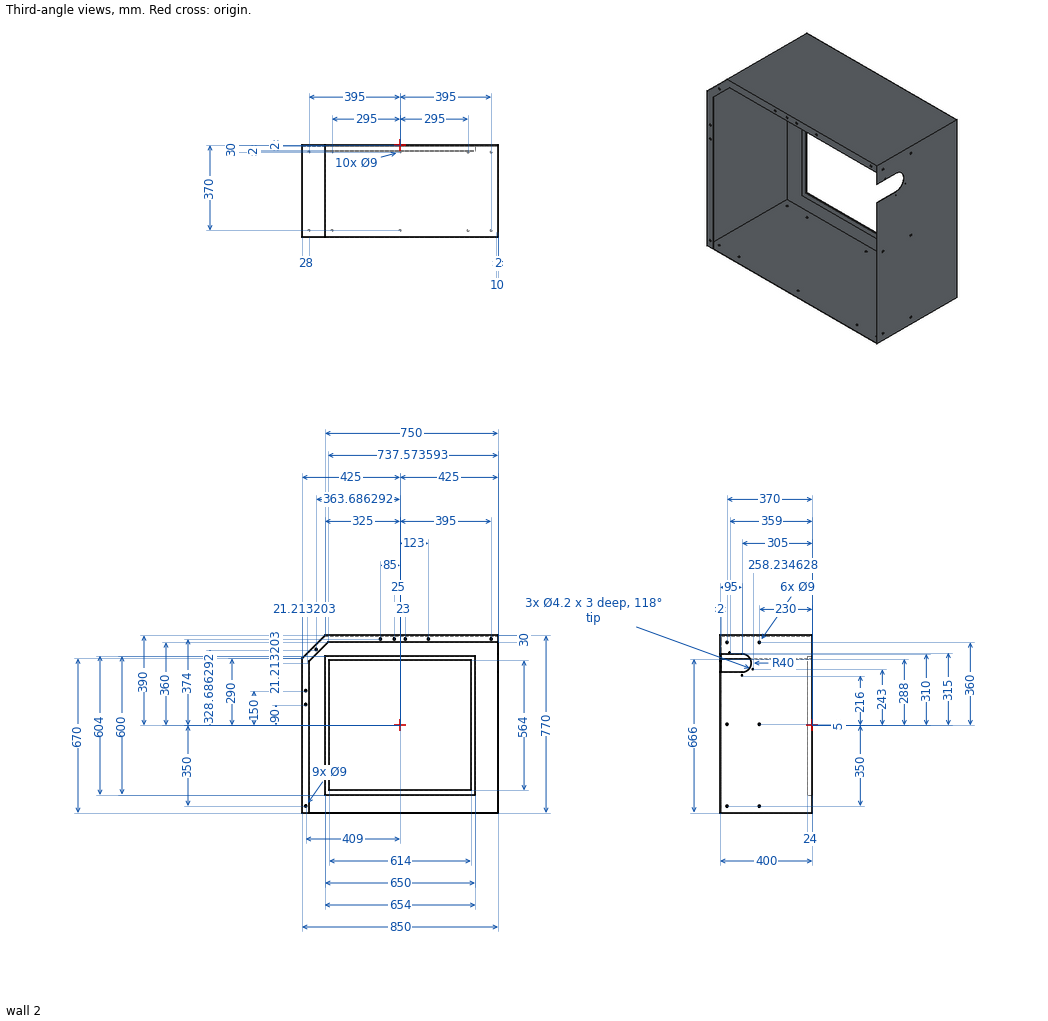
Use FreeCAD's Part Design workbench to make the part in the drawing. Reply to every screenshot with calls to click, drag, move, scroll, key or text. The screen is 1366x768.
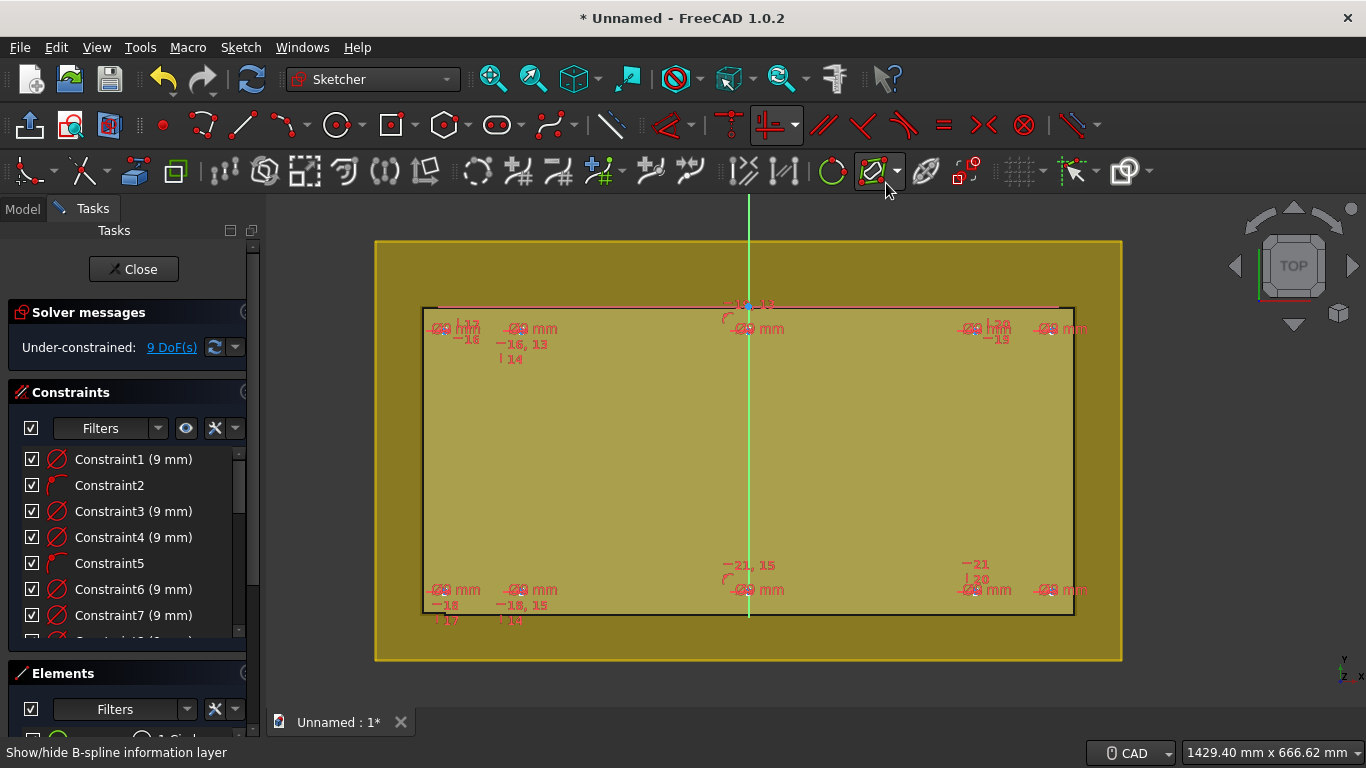
click(976, 592)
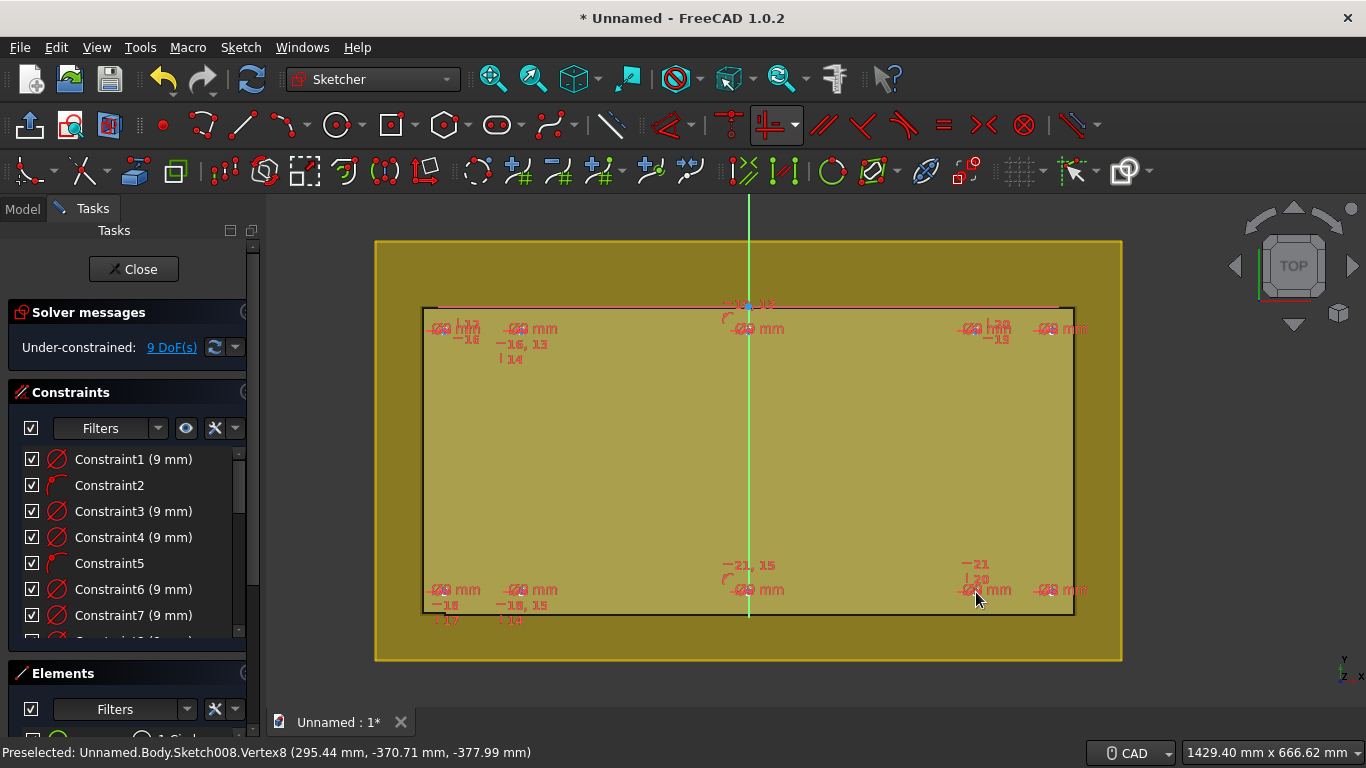
click(1052, 592)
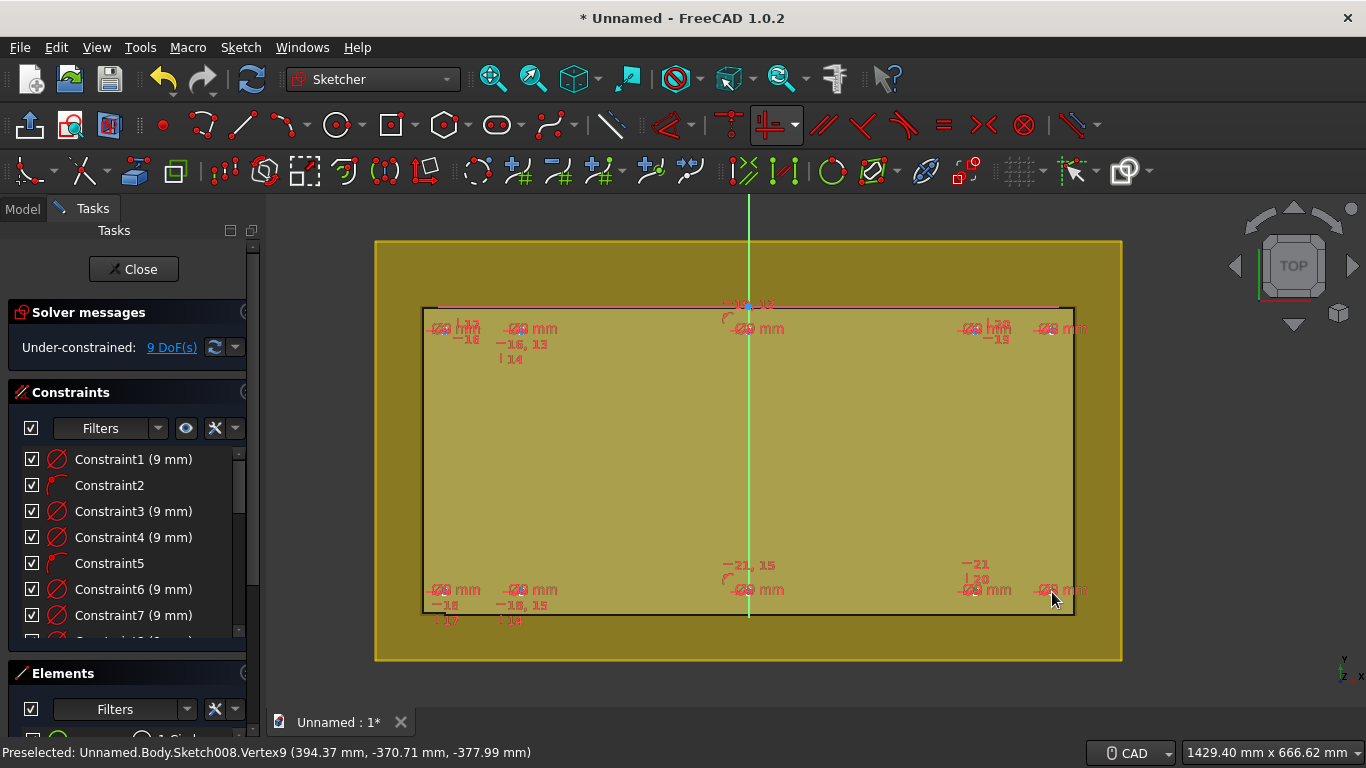
click(798, 126)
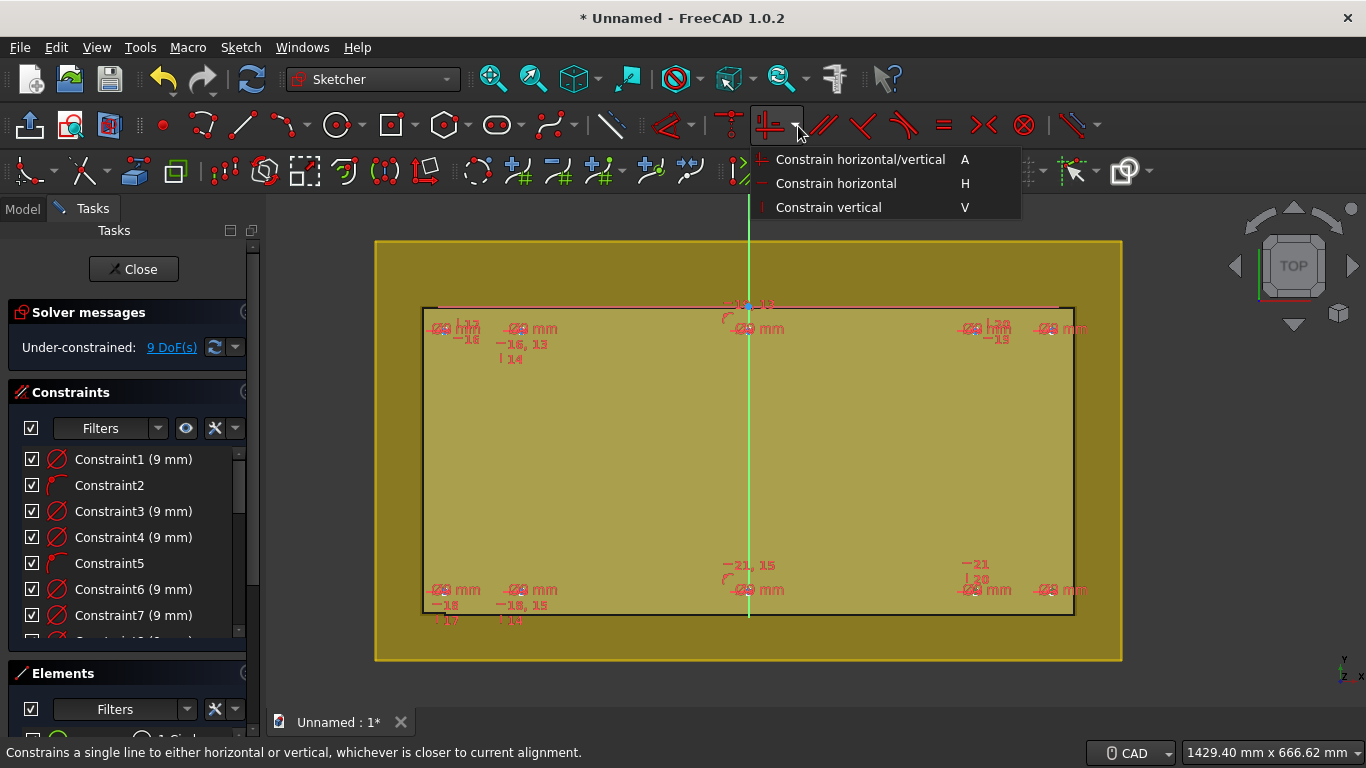
click(886, 183)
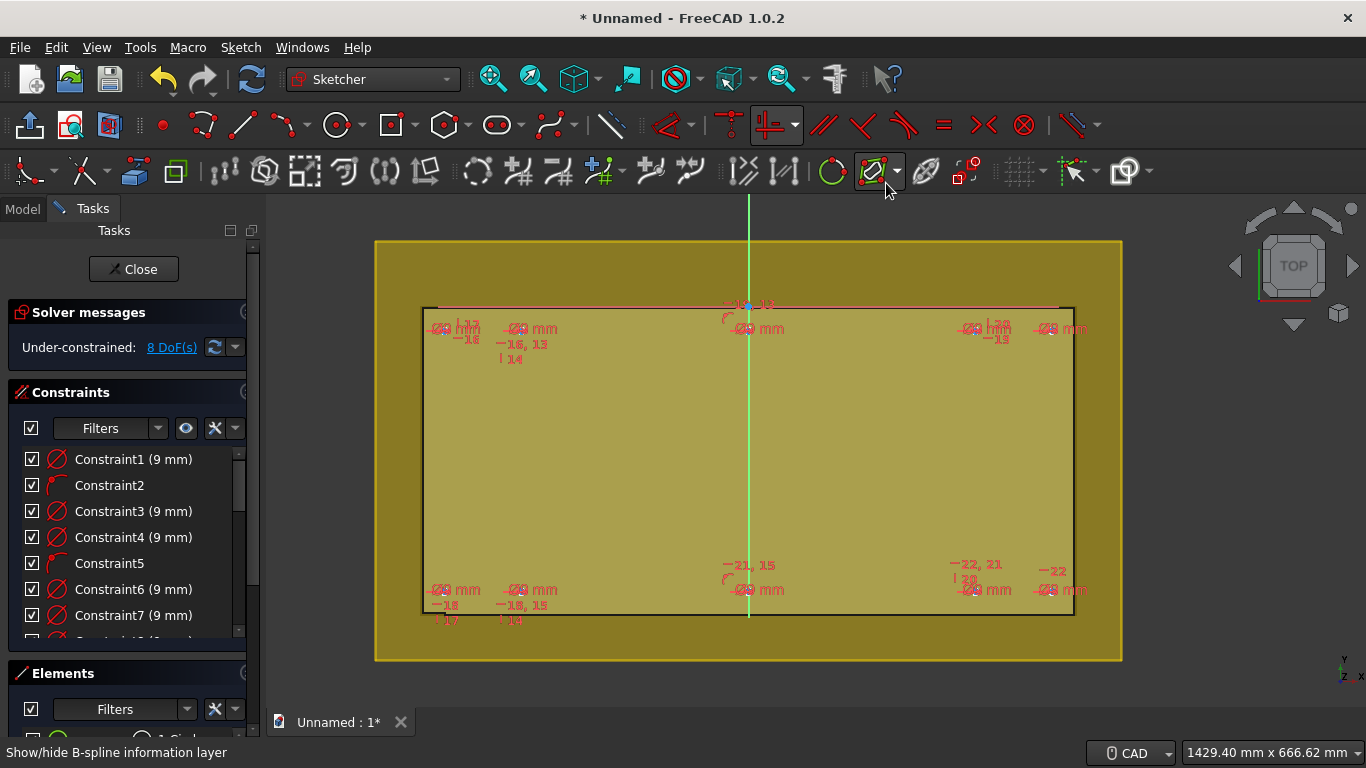
click(1052, 592)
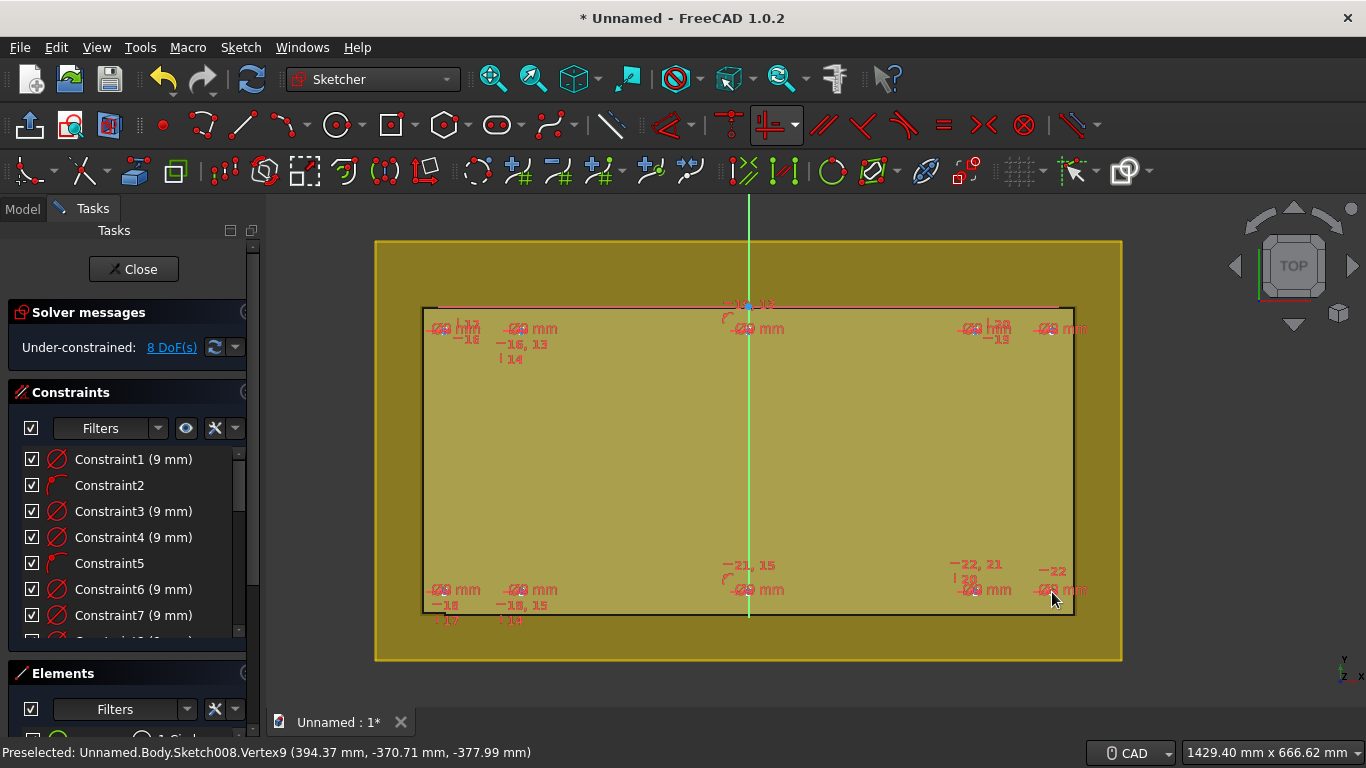
click(1052, 331)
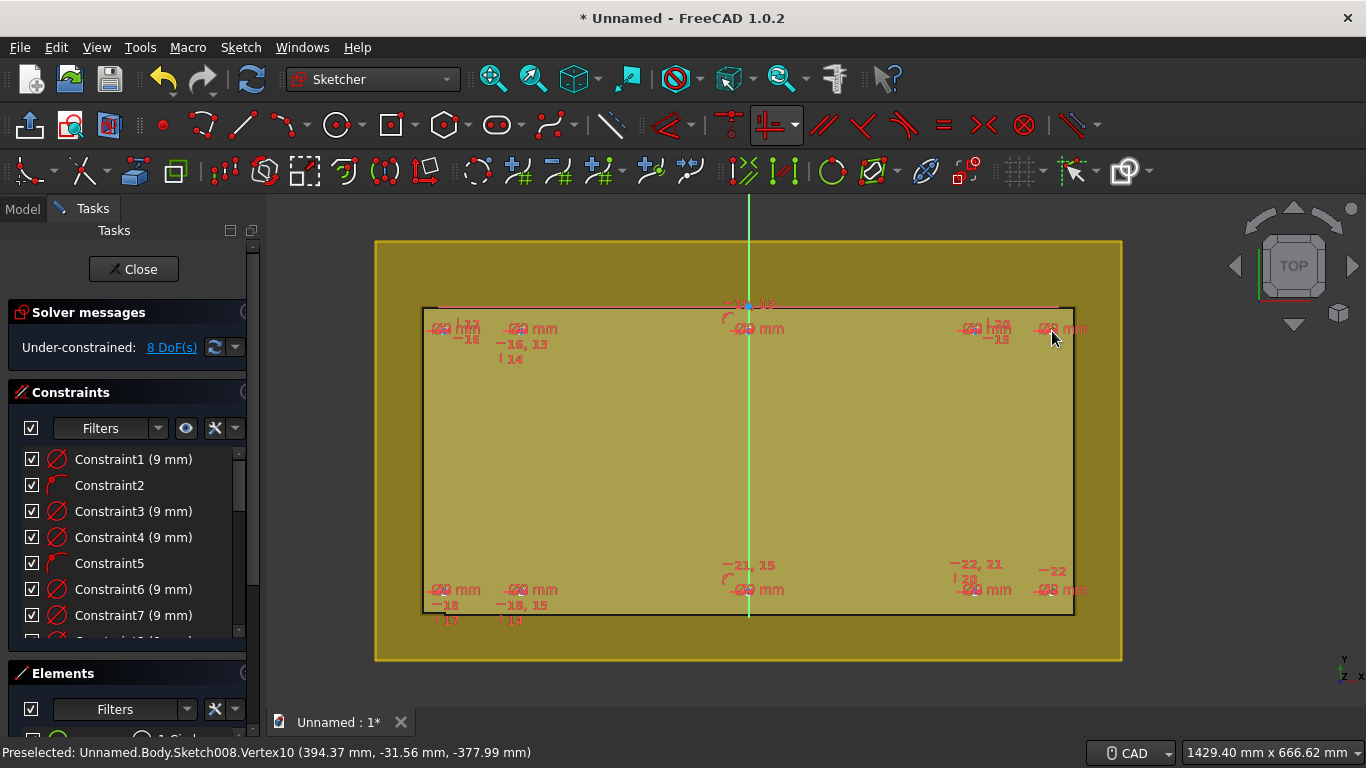
key(v)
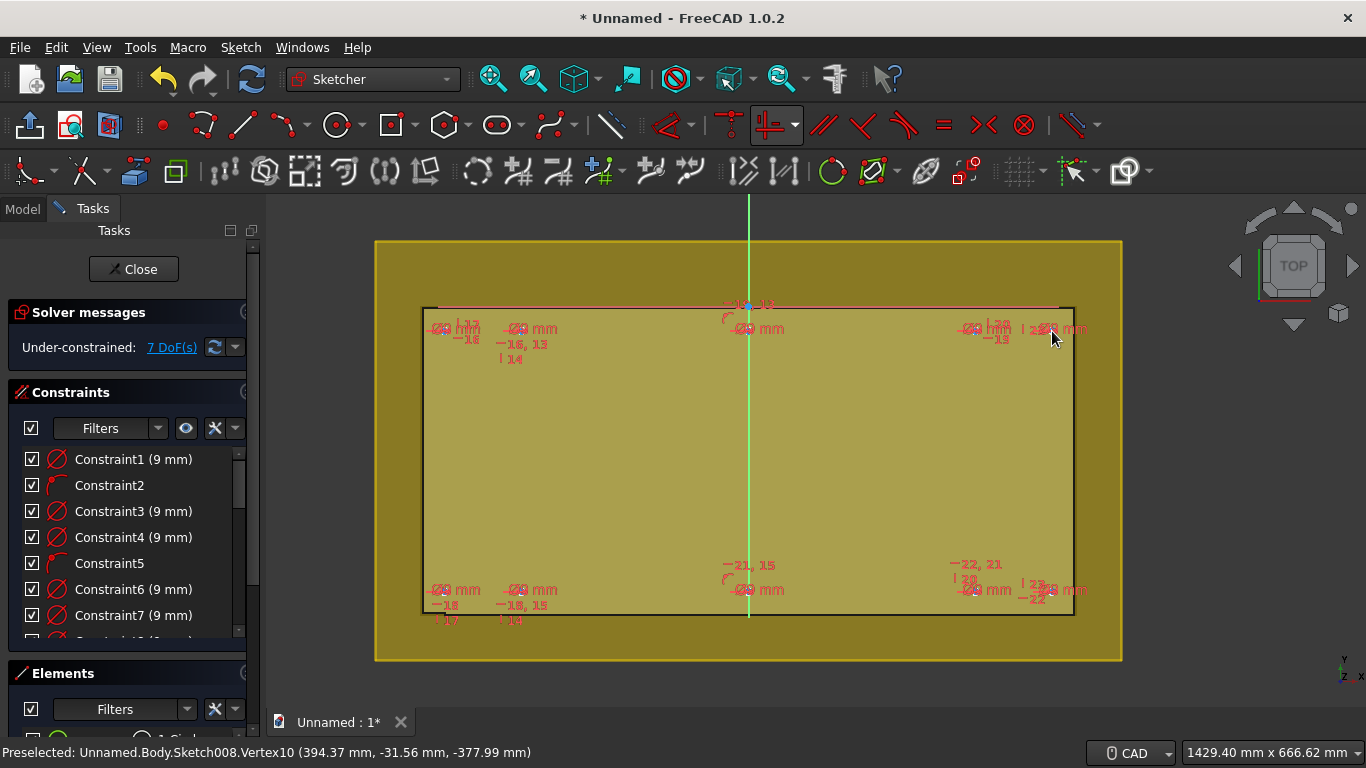
click(976, 331)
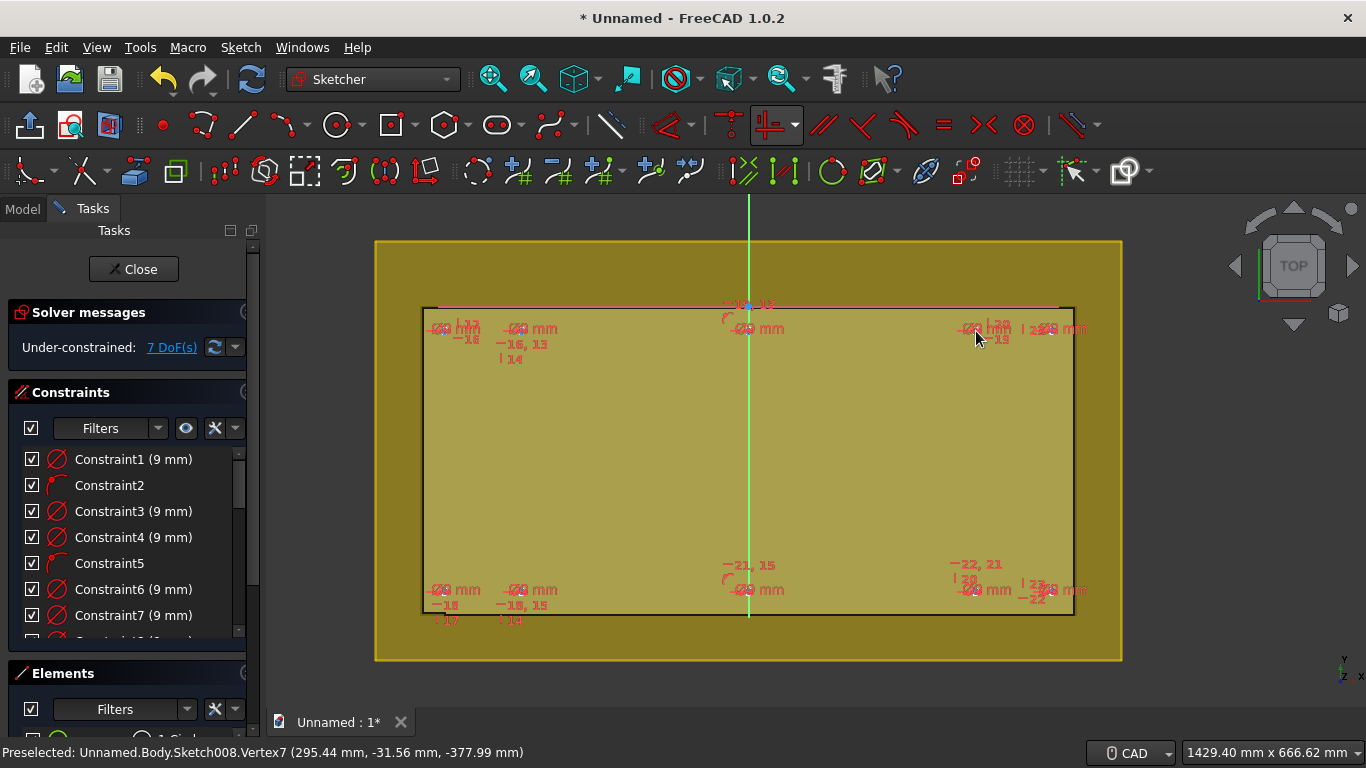
click(1052, 331)